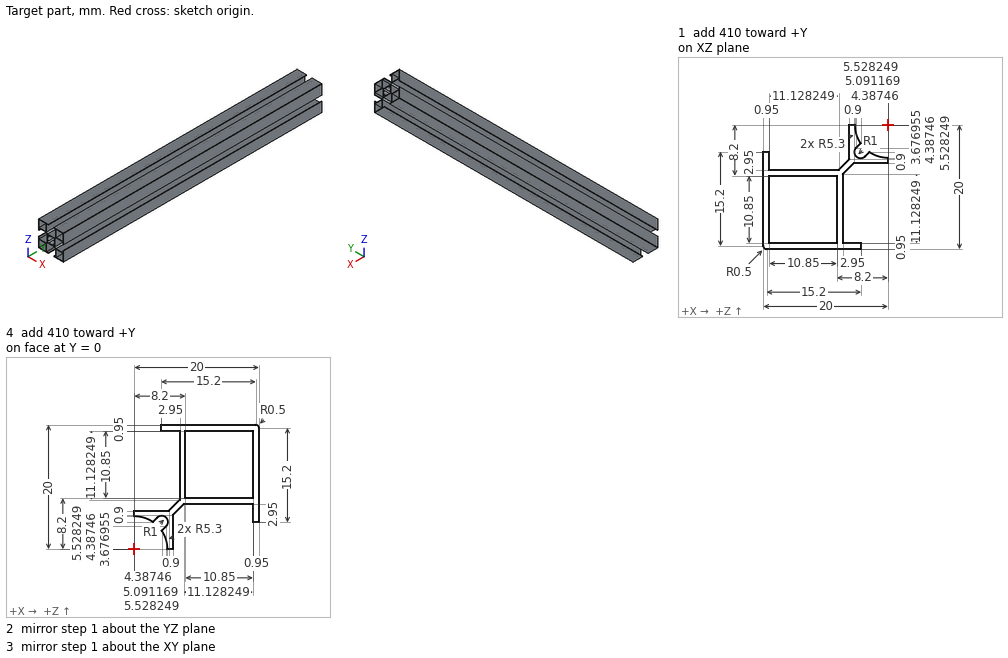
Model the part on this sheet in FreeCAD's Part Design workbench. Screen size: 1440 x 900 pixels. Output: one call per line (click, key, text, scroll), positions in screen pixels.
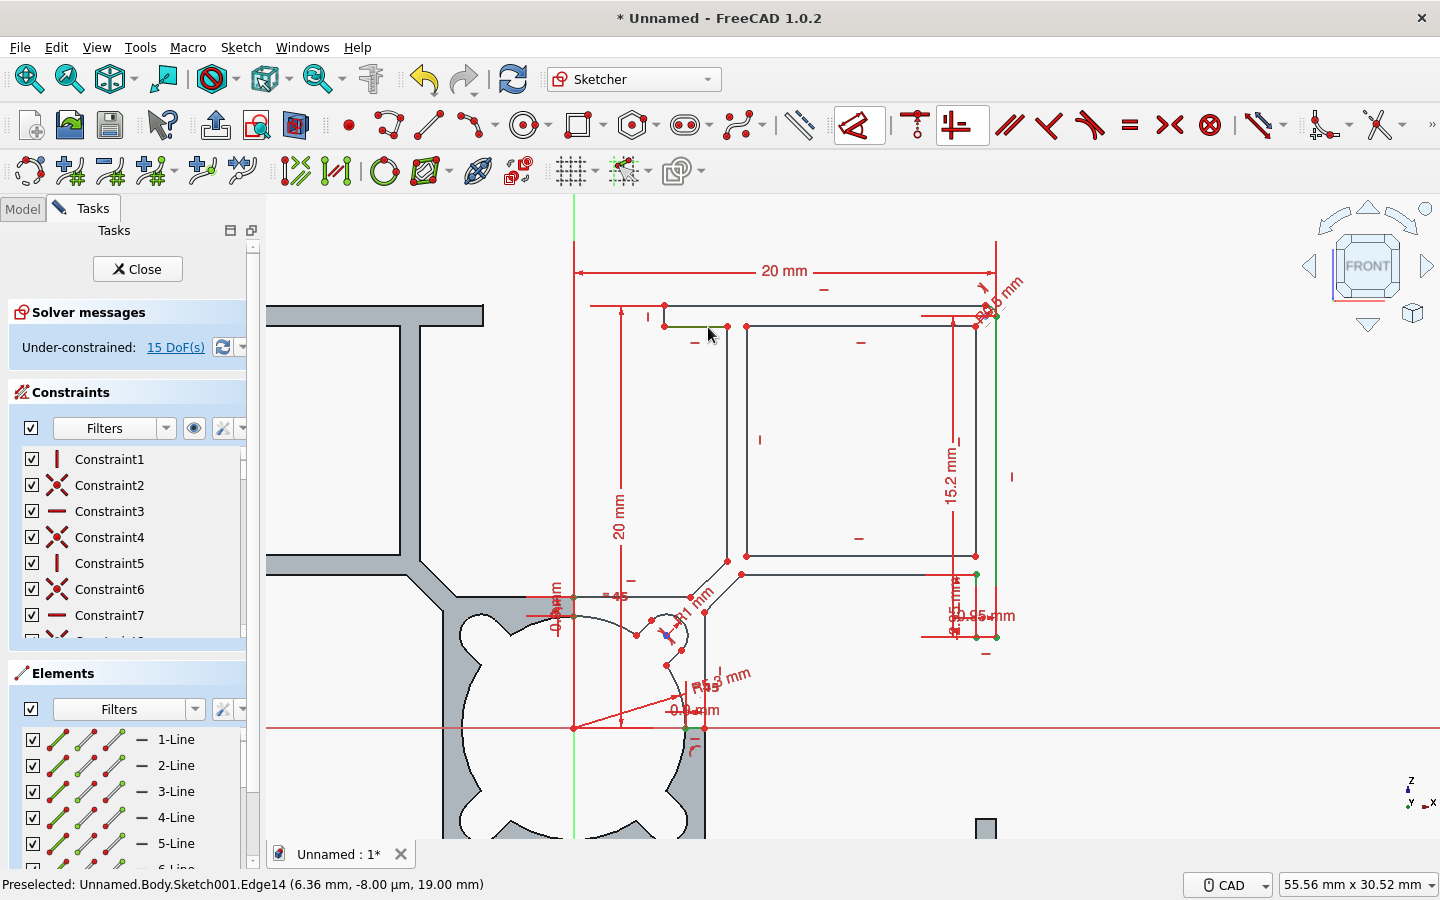
key(l)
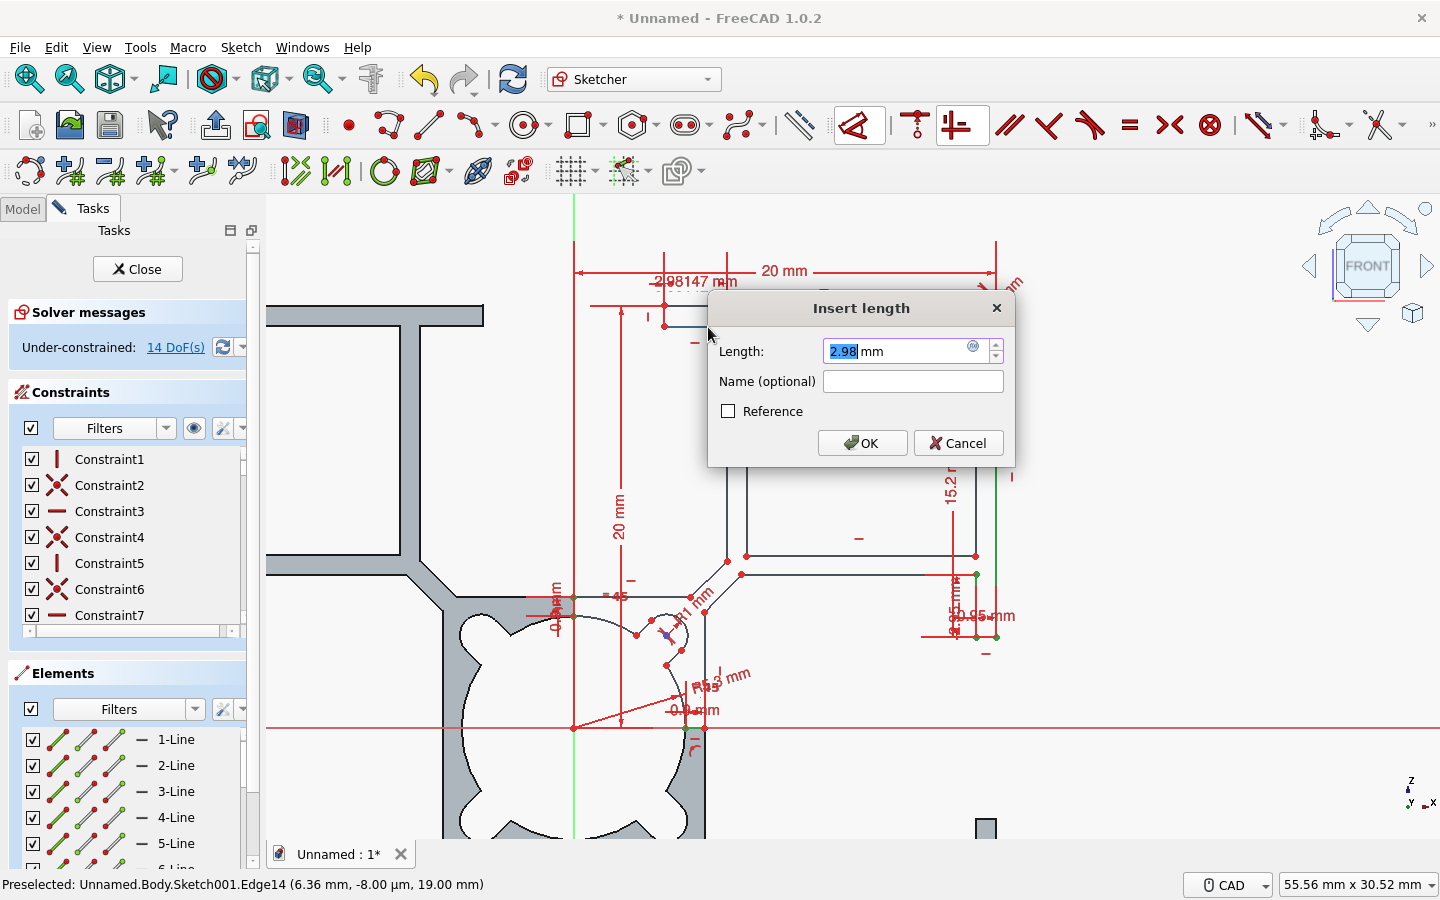
text(2.95)
key(Return)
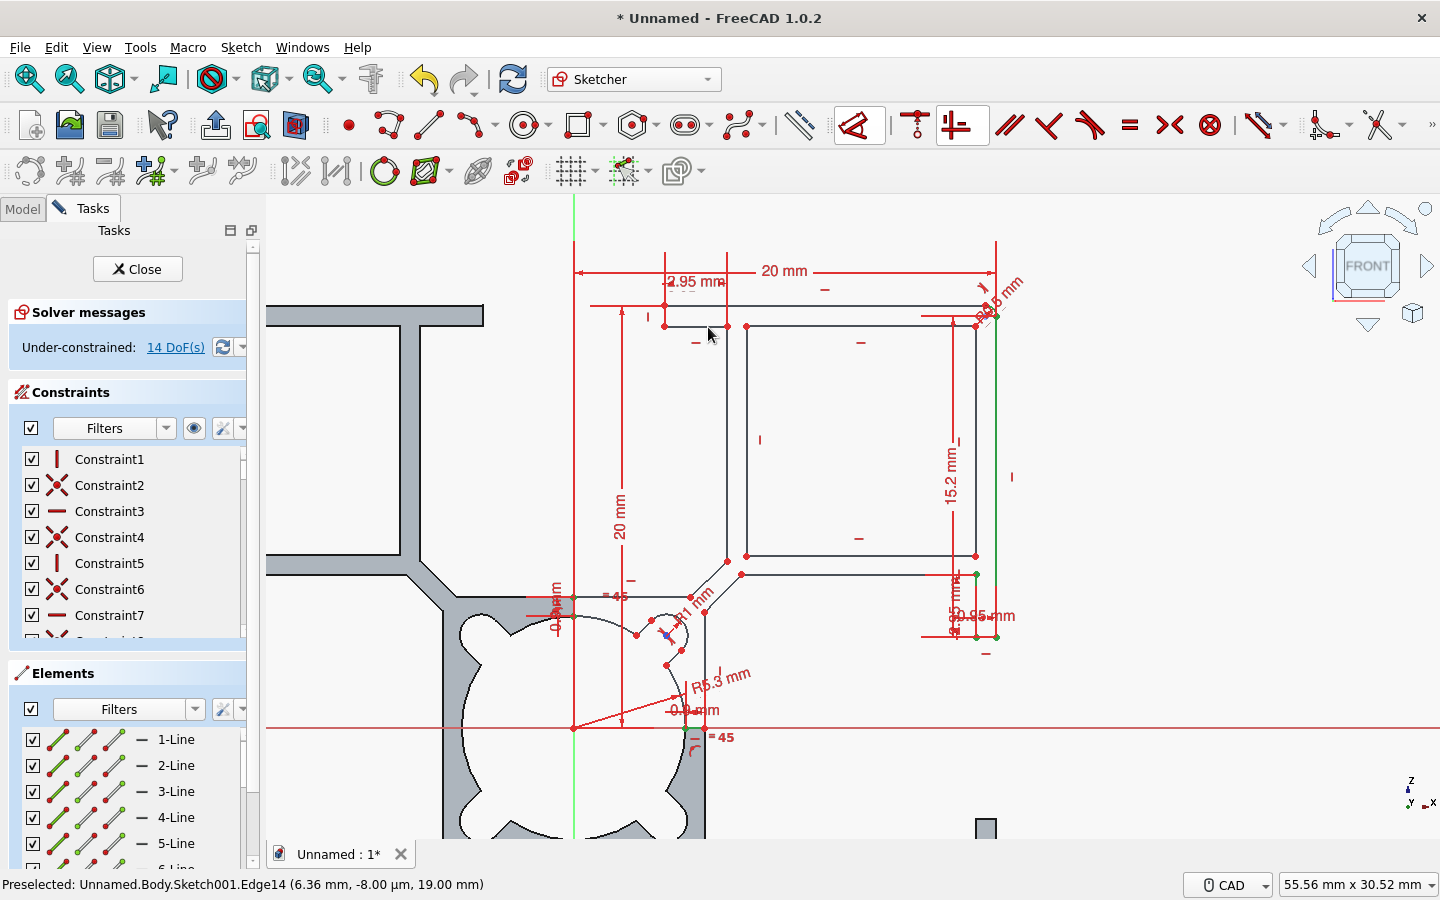
scroll(665, 316, up, 4)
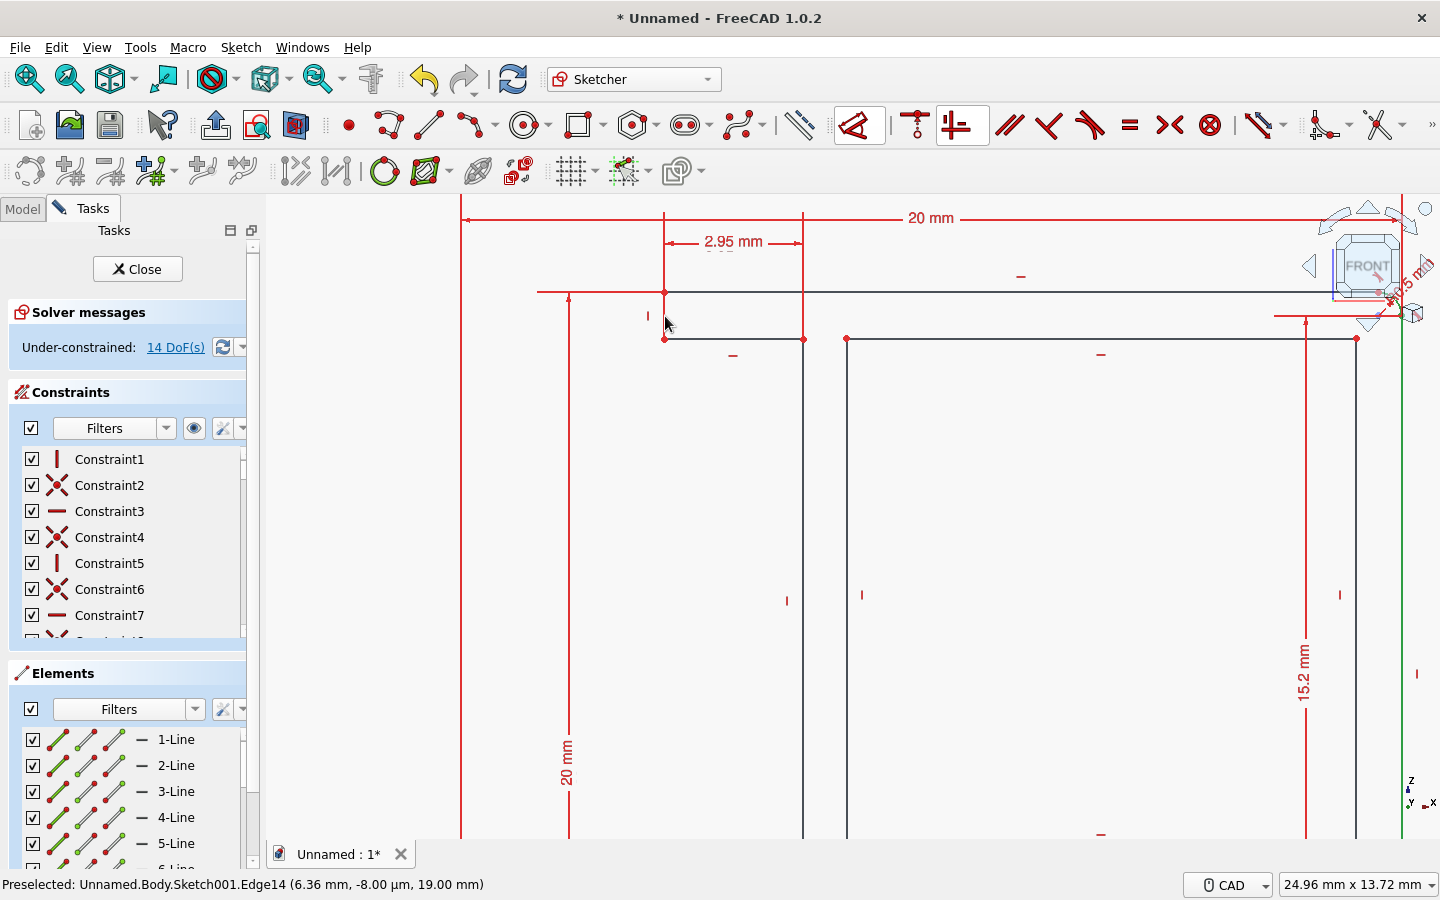
click(664, 316)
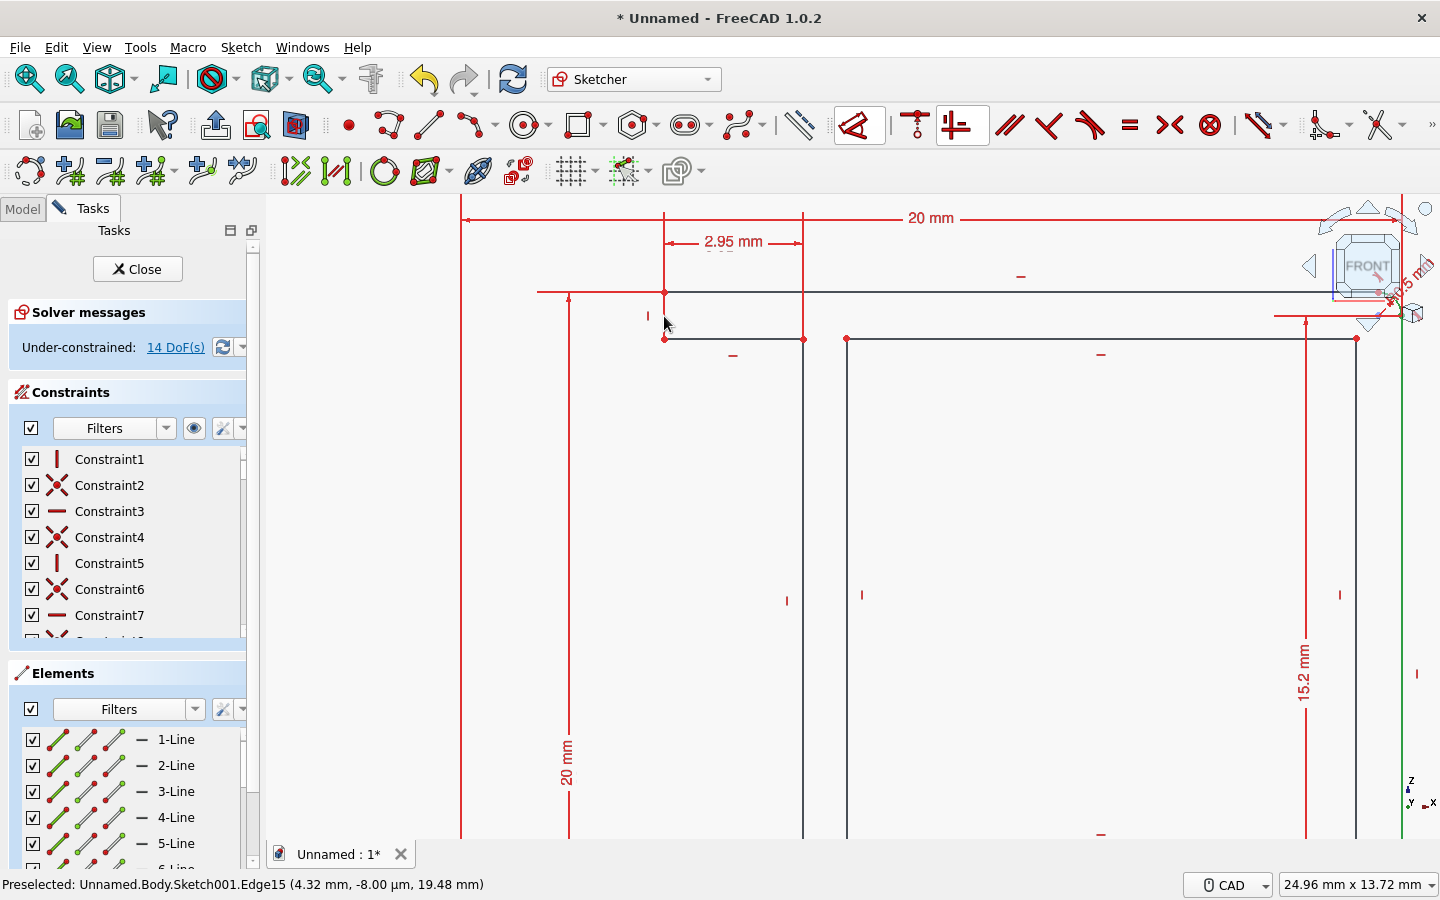
click(880, 126)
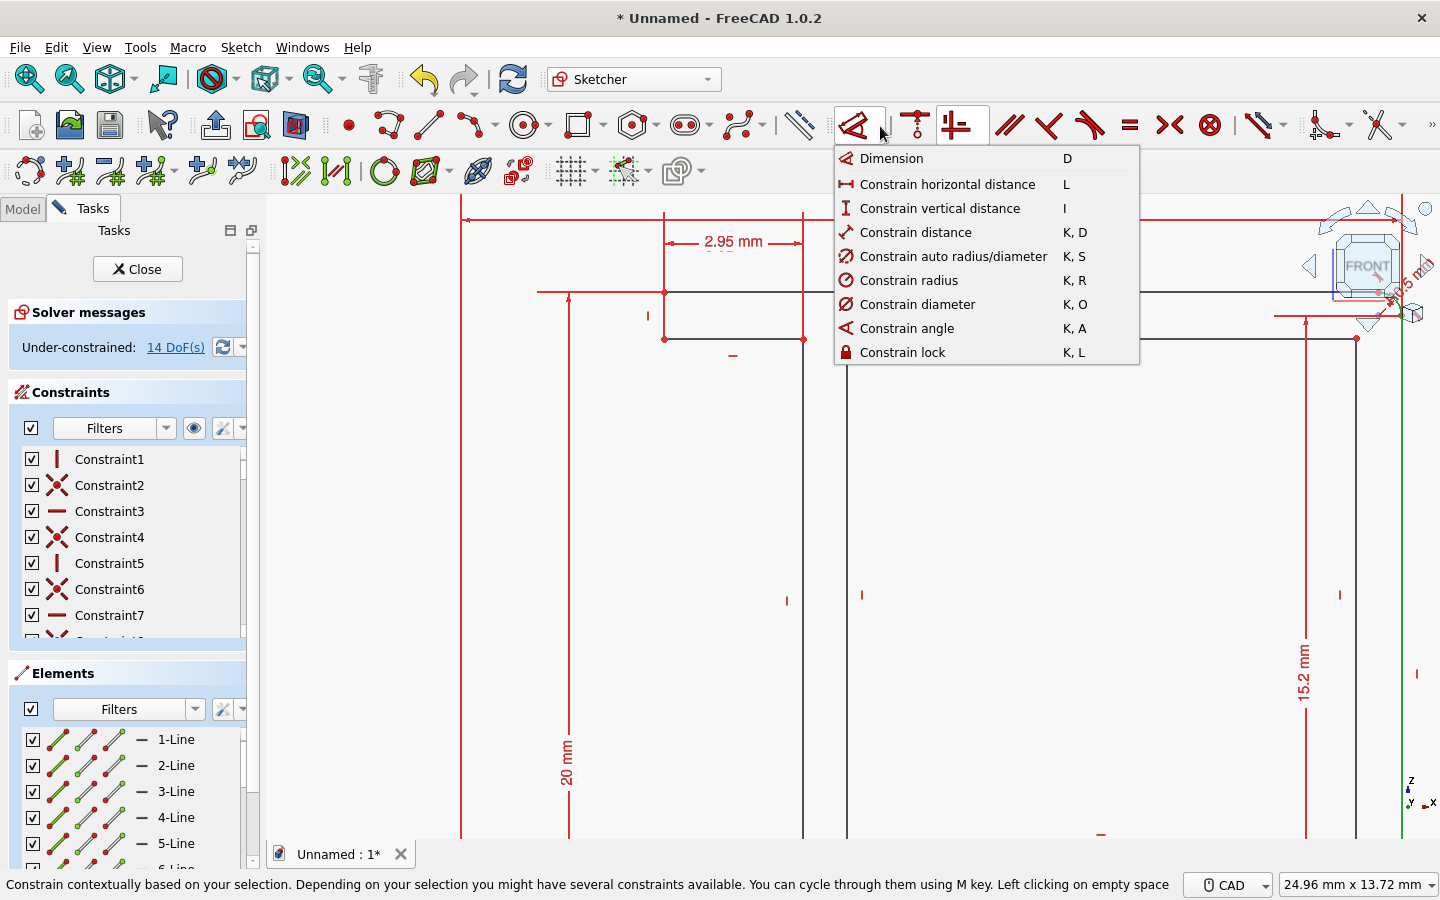
click(987, 208)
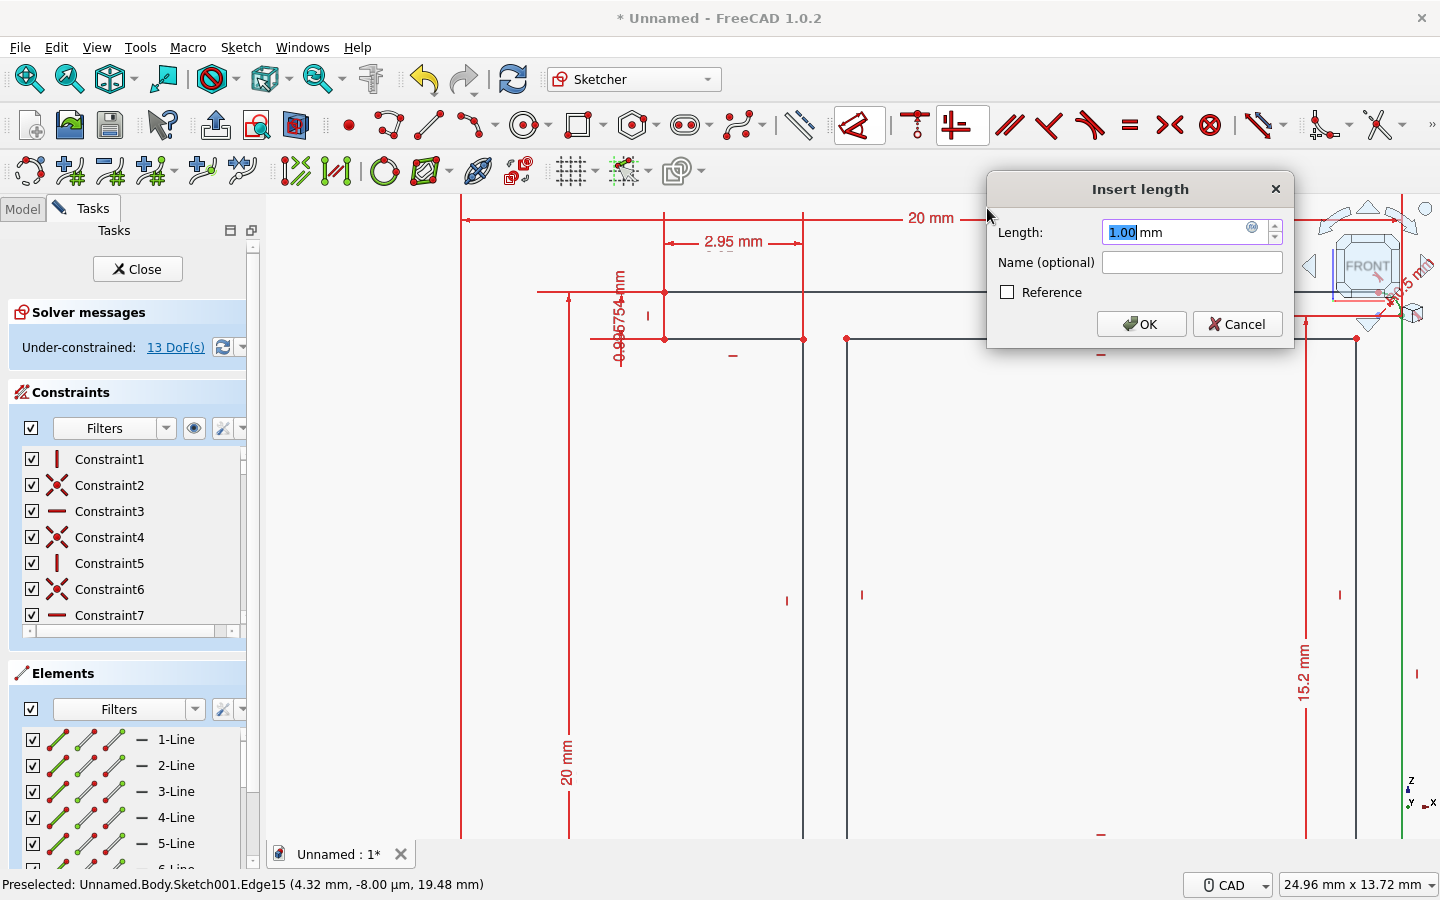
text(0.95)
key(Return)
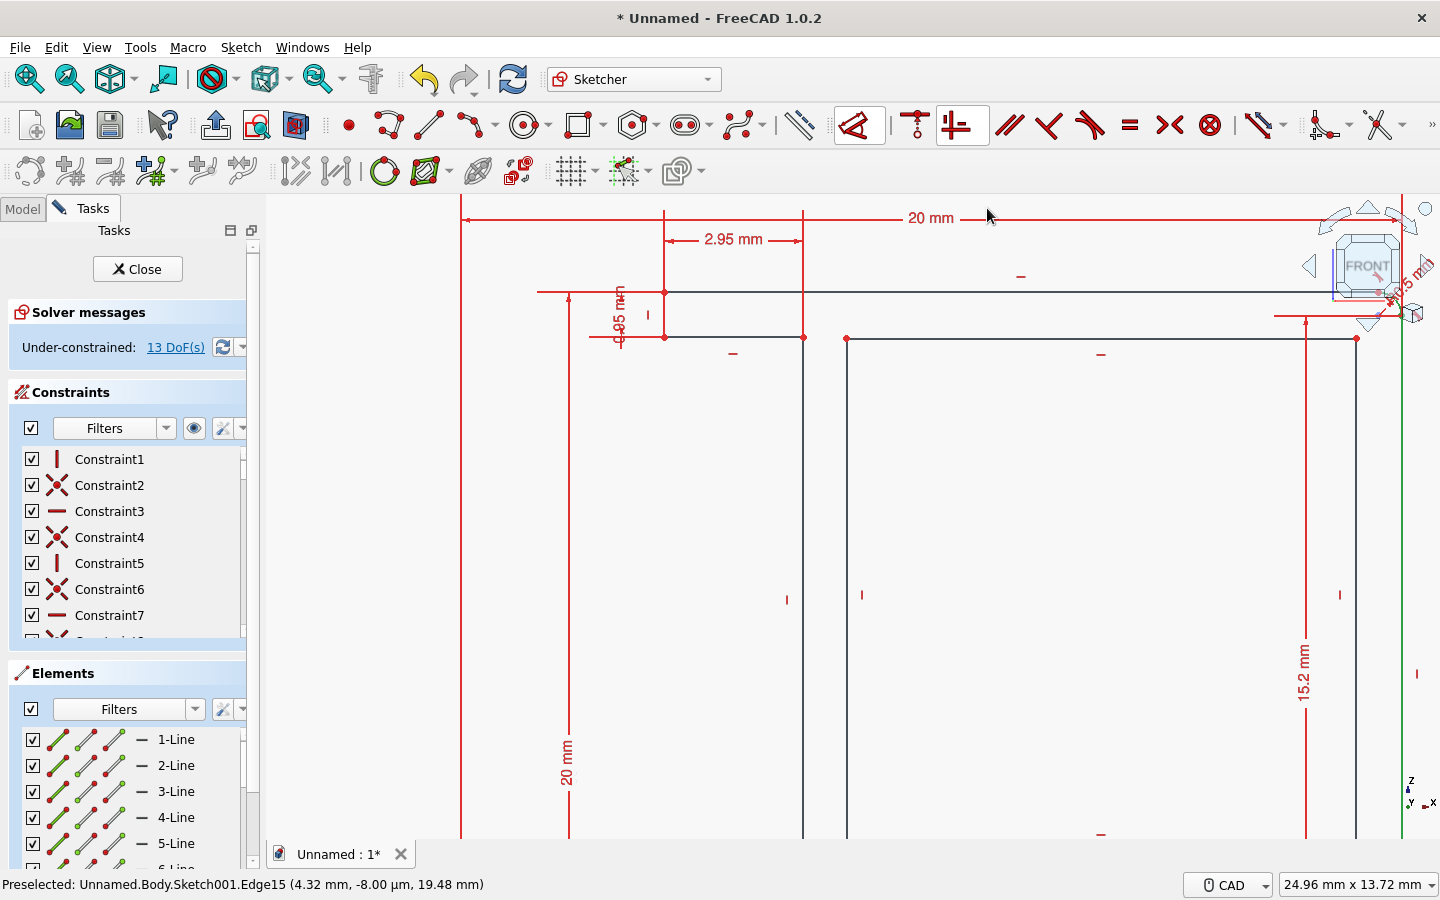
click(879, 292)